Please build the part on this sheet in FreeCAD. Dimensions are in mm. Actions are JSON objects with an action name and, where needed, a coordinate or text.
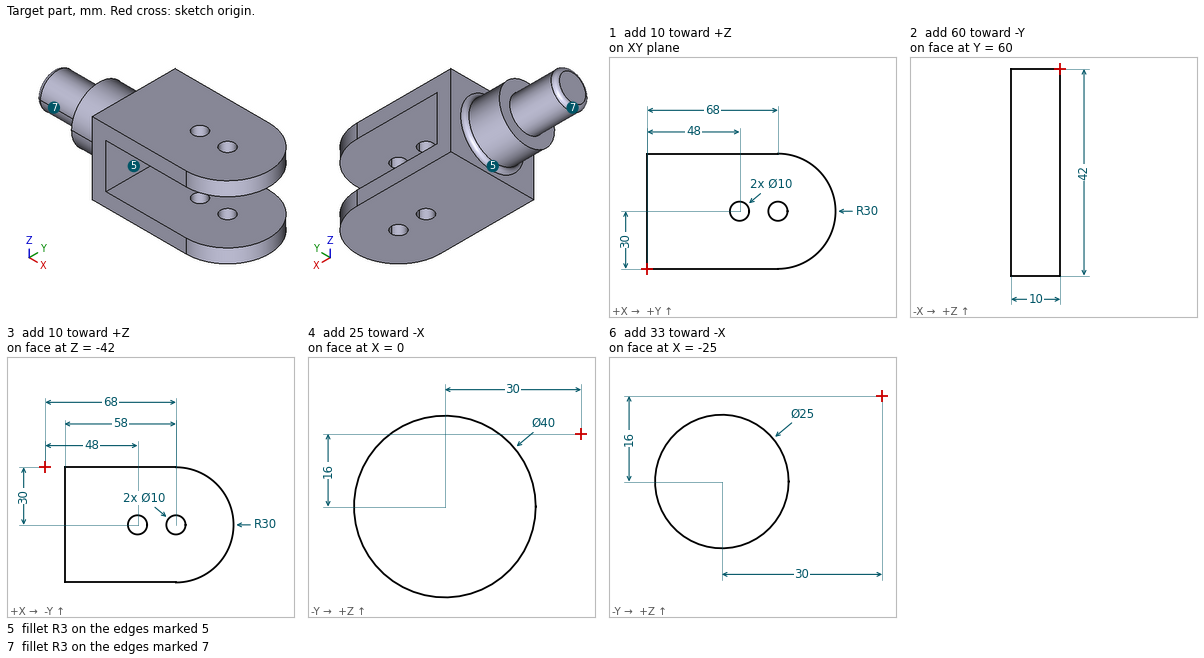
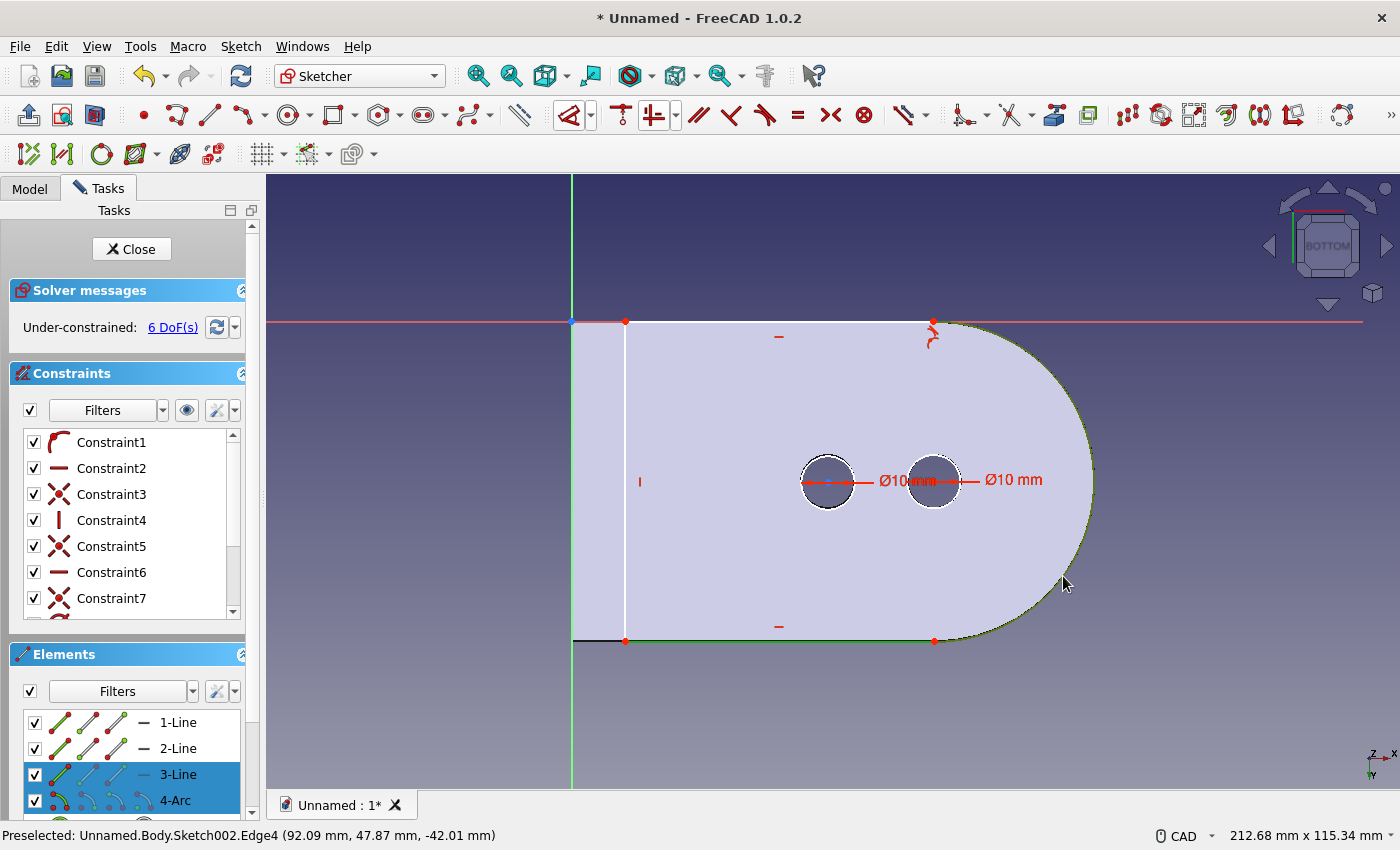
{"action": "key", "text": "t"}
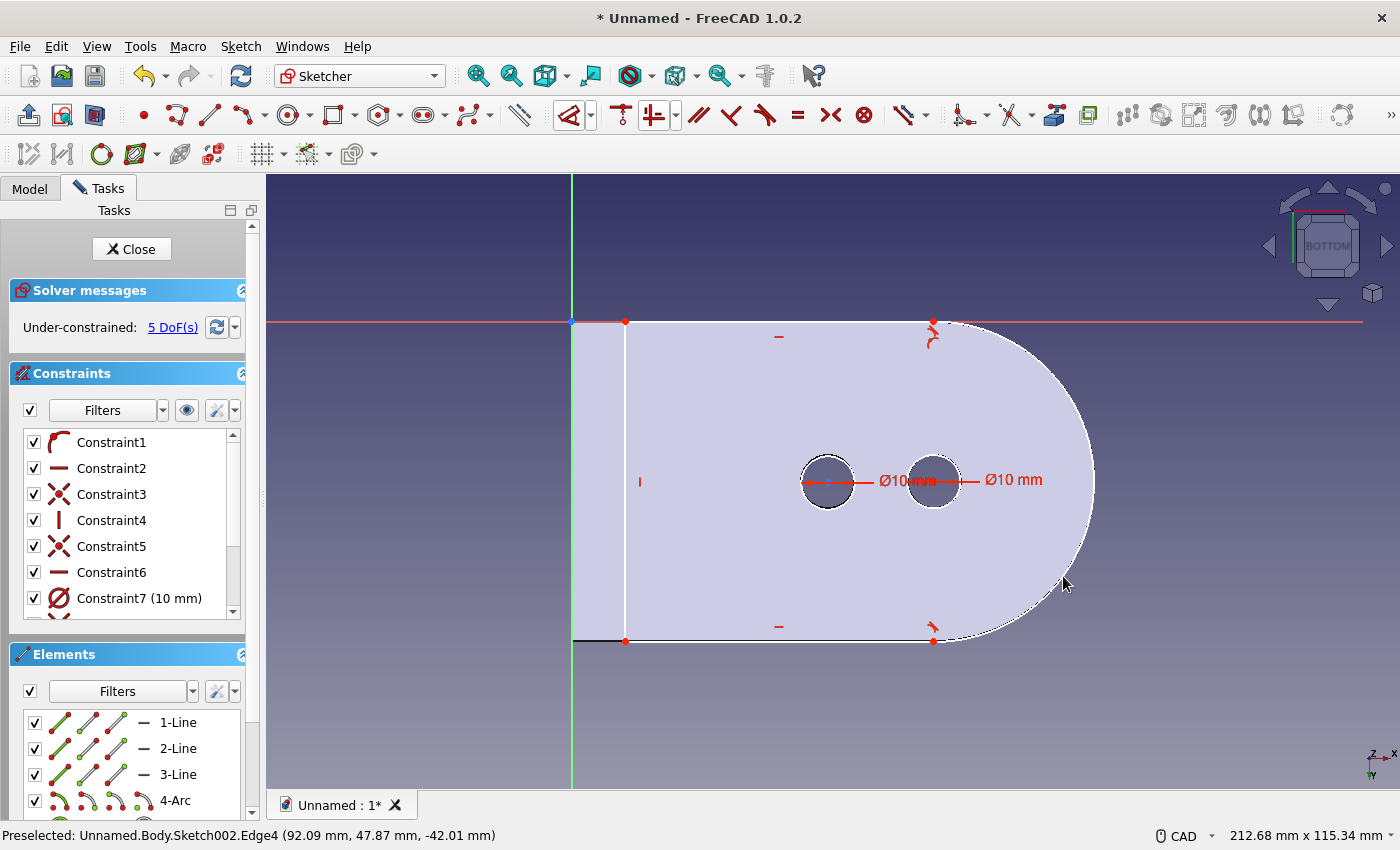
{"action": "left_click", "coordinate": [568, 116]}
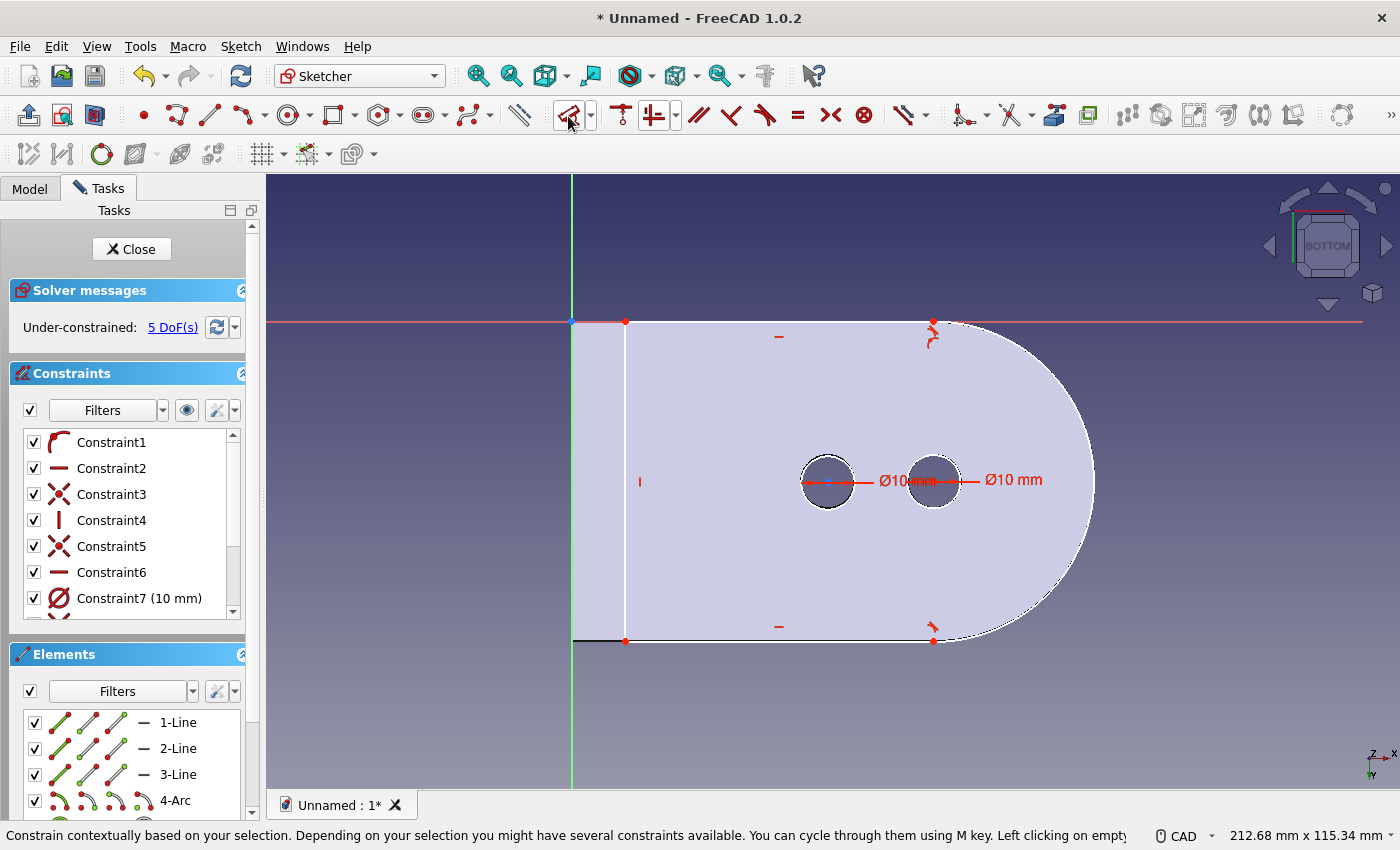
{"action": "left_click", "coordinate": [1063, 576]}
{"action": "left_click", "coordinate": [1089, 595]}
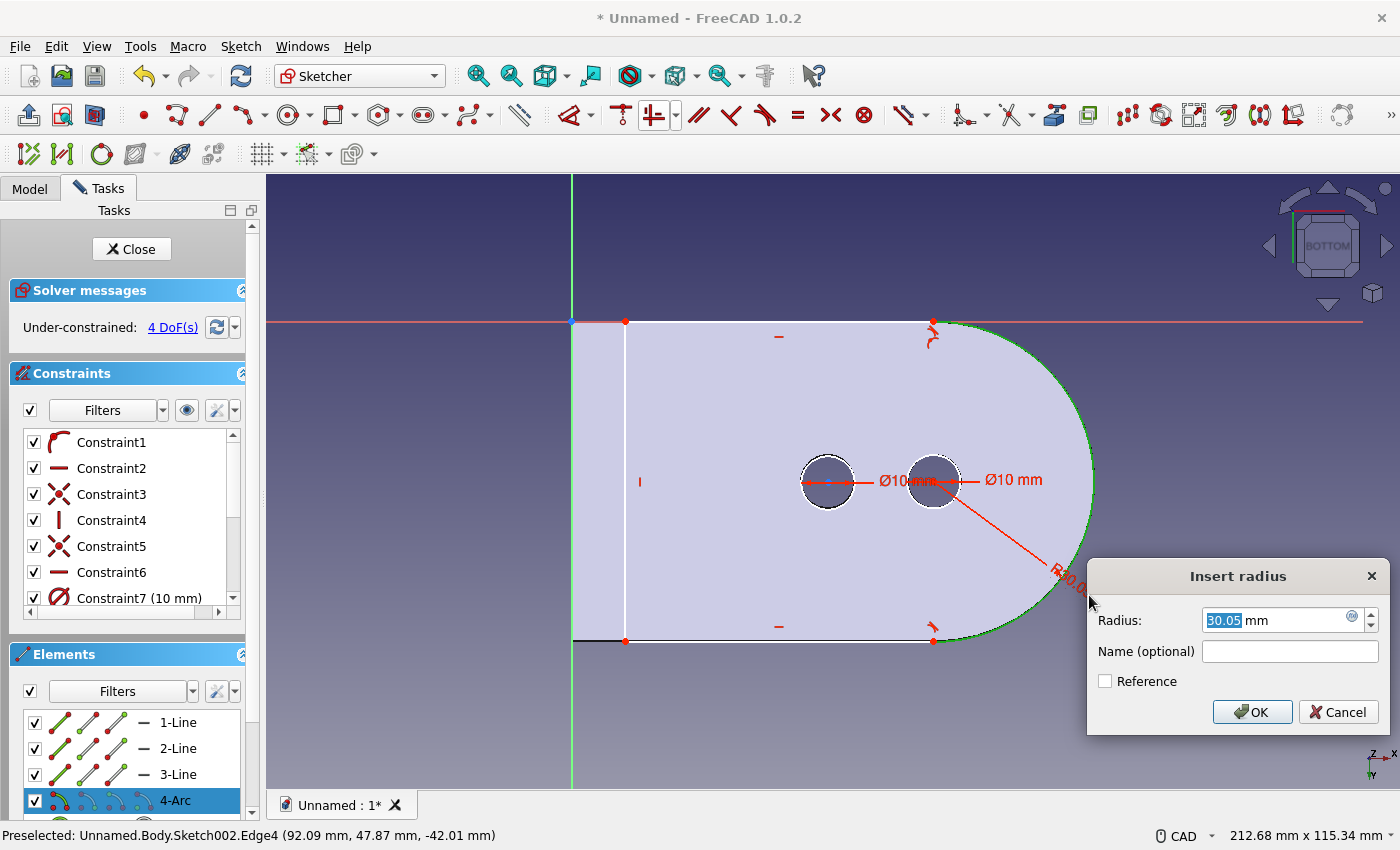
{"action": "type", "text": "30"}
{"action": "key", "text": "Return"}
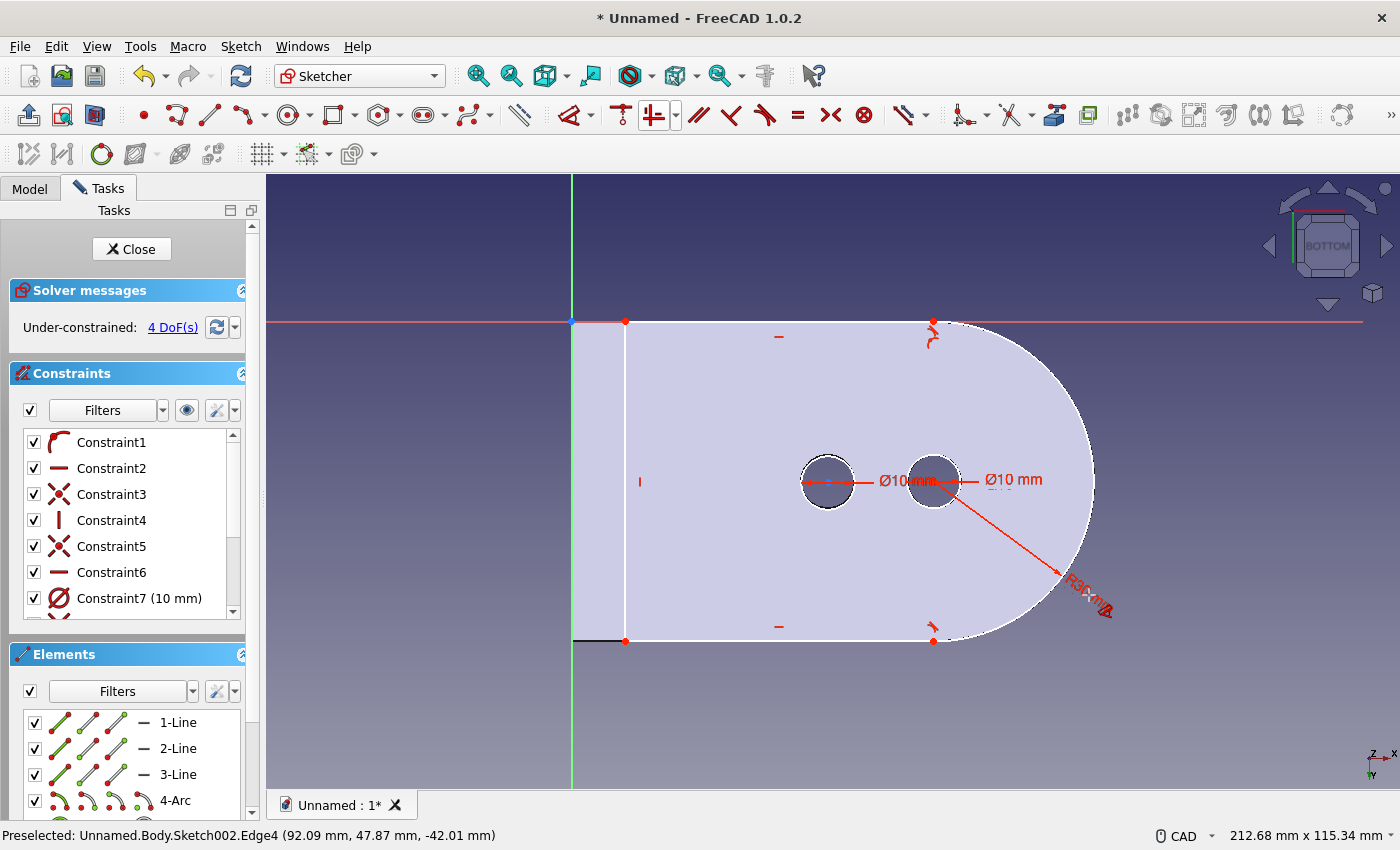
{"action": "left_click", "coordinate": [841, 322]}
{"action": "left_click", "coordinate": [779, 288]}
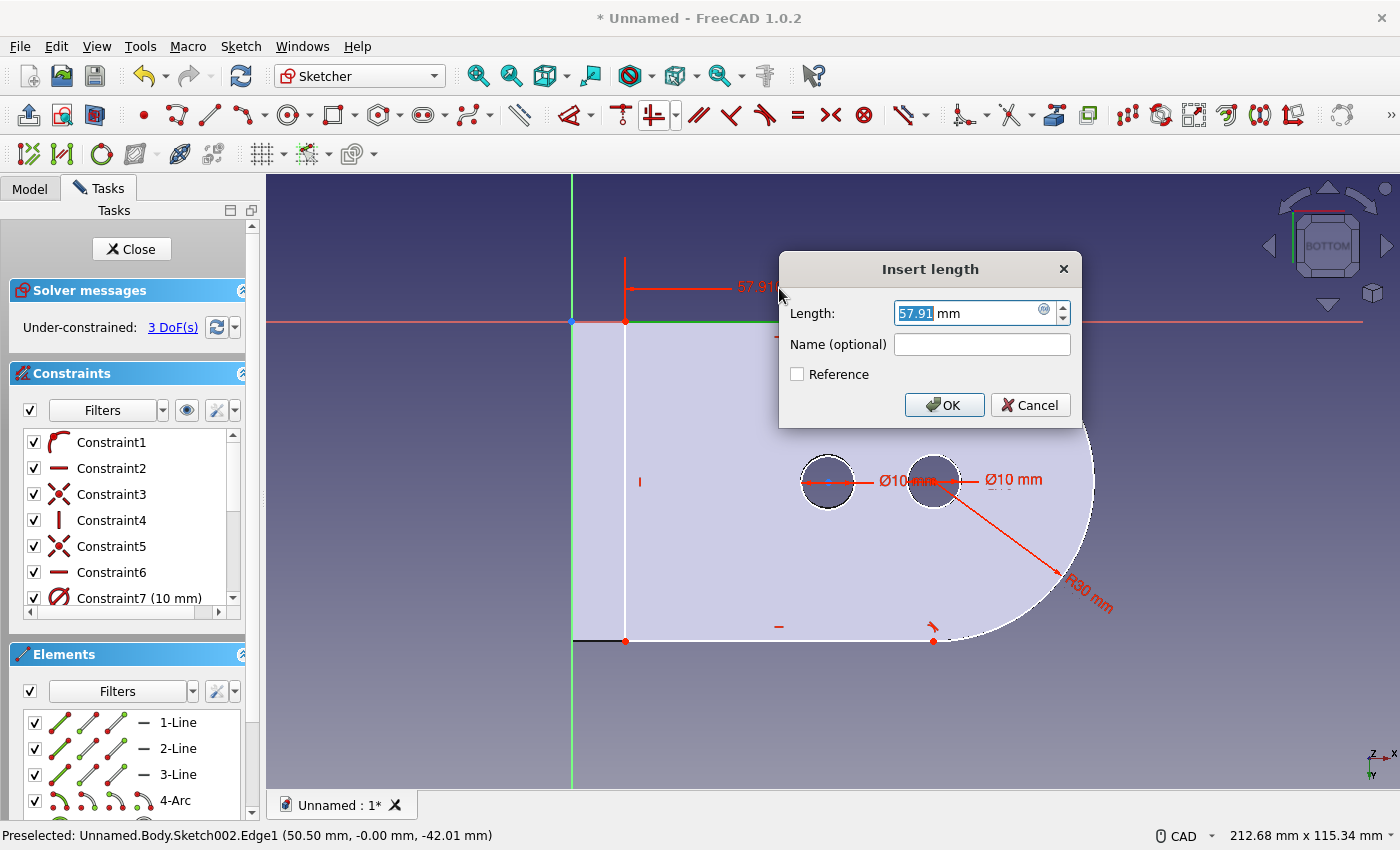
{"action": "type", "text": "58"}
{"action": "key", "text": "Return"}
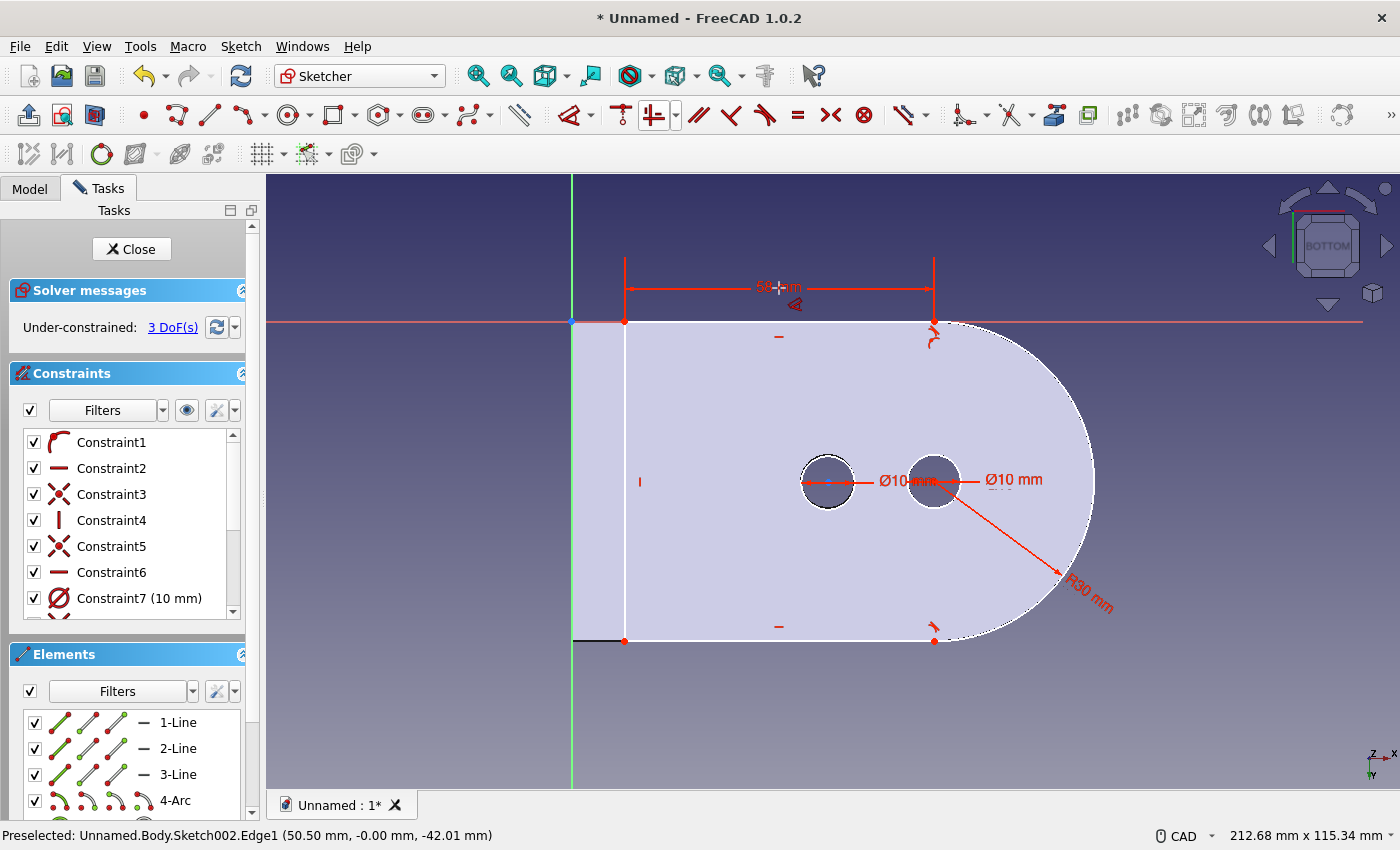
{"action": "left_click", "coordinate": [934, 482]}
{"action": "left_click", "coordinate": [670, 288]}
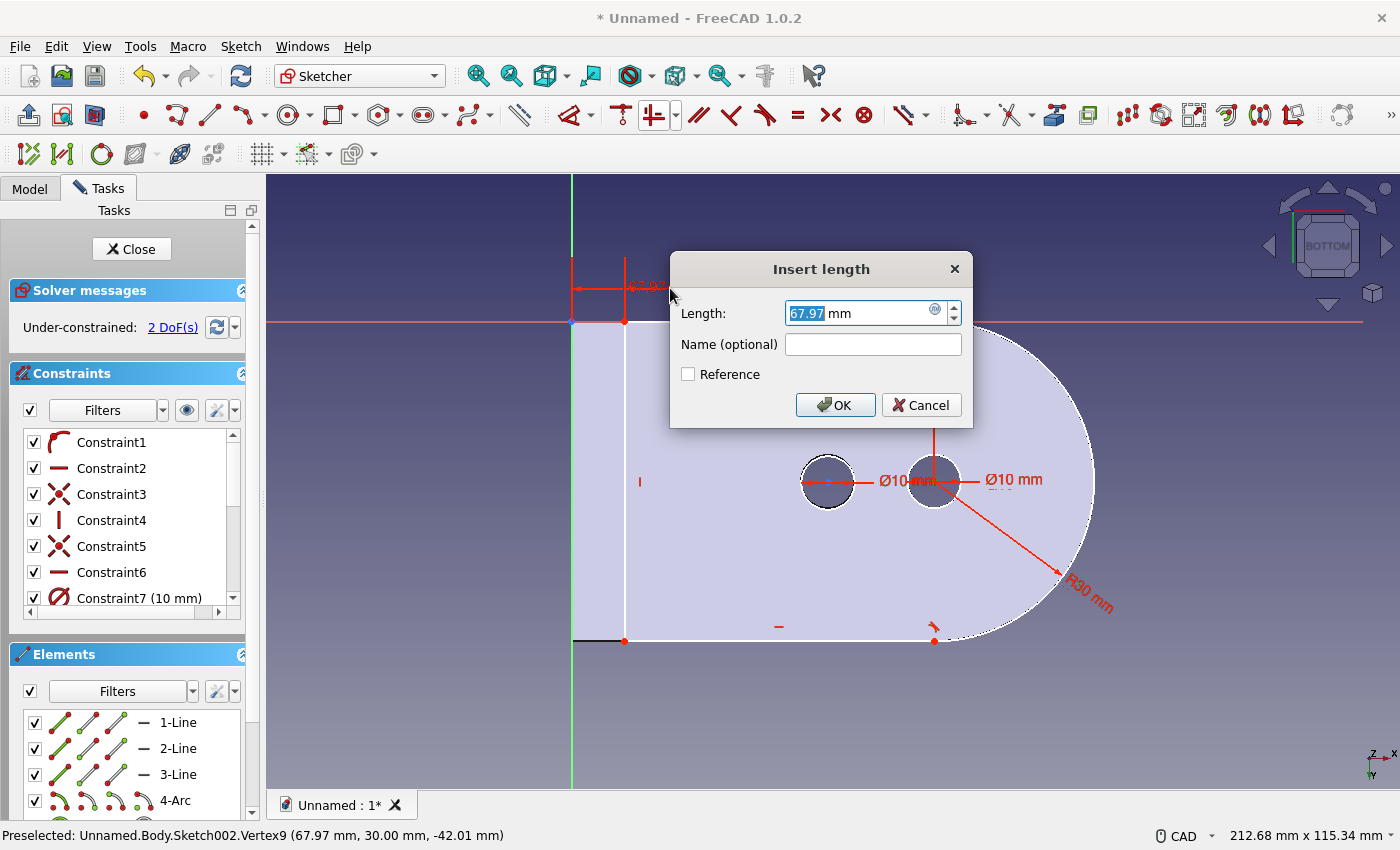
{"action": "type", "text": "68"}
{"action": "key", "text": "Return"}